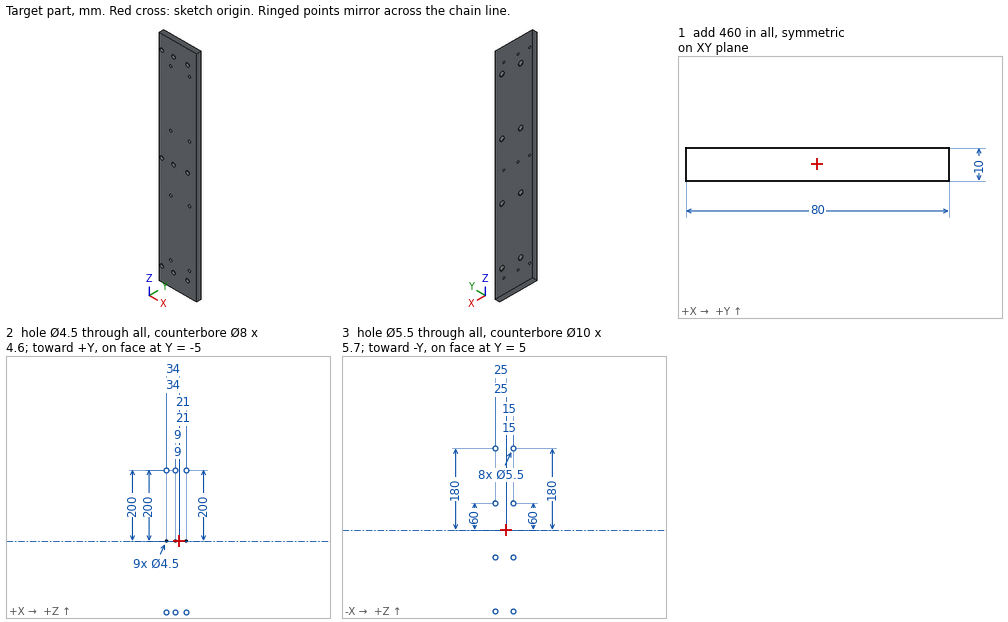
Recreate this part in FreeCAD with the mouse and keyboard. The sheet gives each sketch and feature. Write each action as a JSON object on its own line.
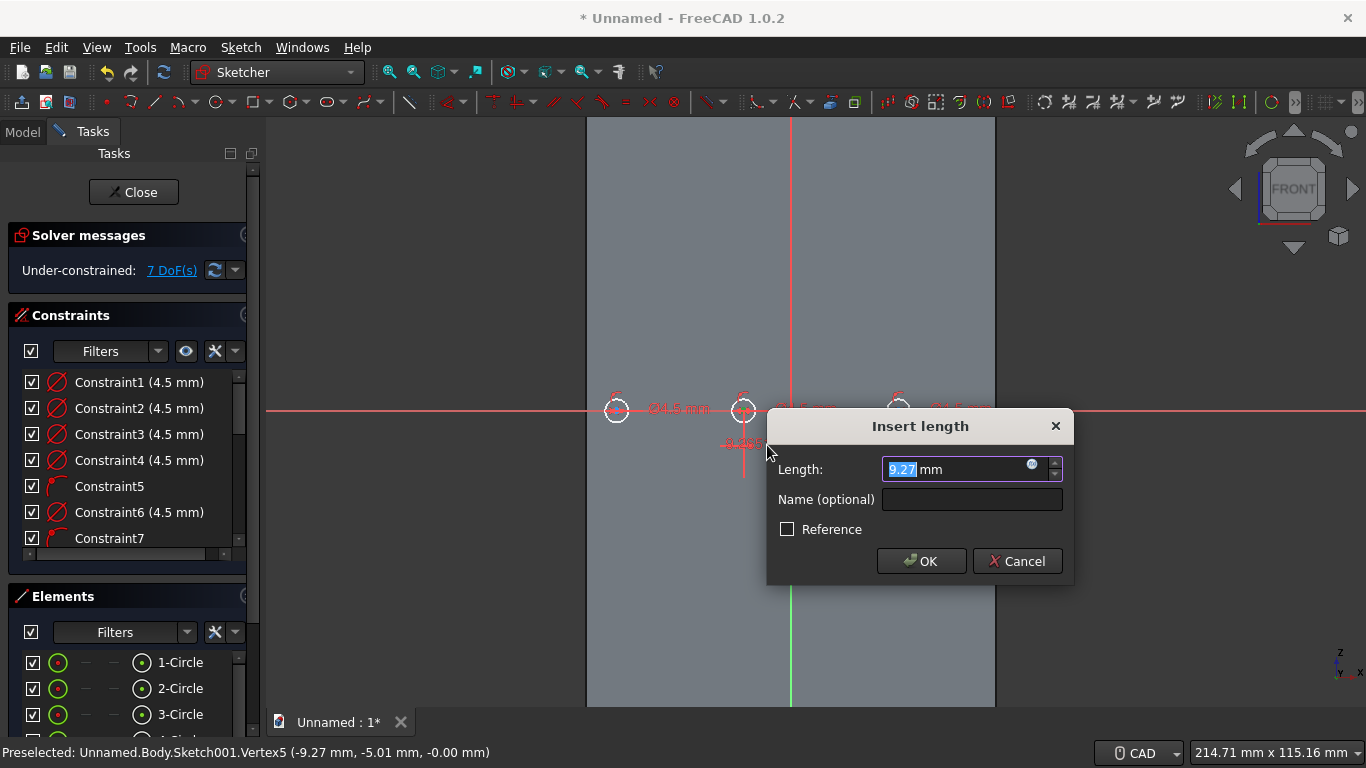
{"action": "type", "text": "9"}
{"action": "key", "text": "Return"}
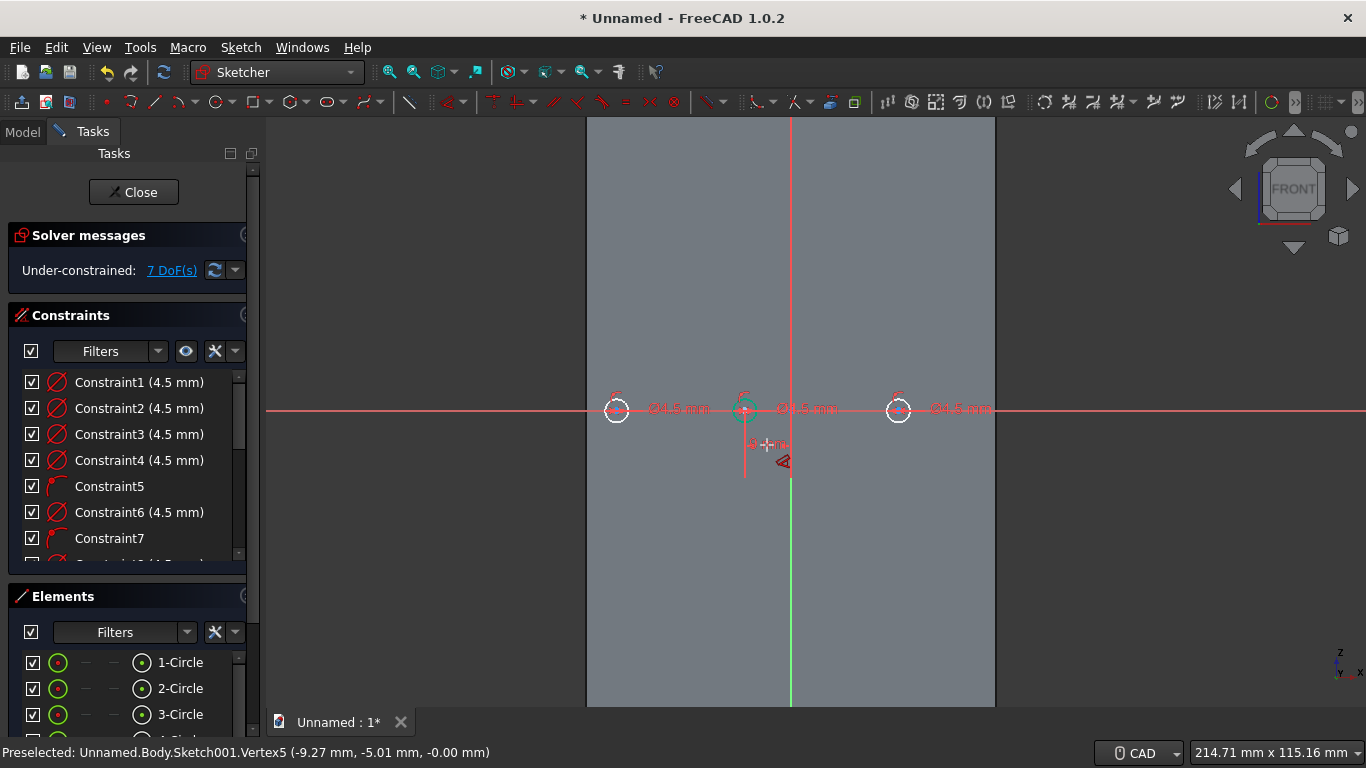
{"action": "scroll", "coordinate": [745, 412], "scroll_direction": "down", "scroll_amount": 9}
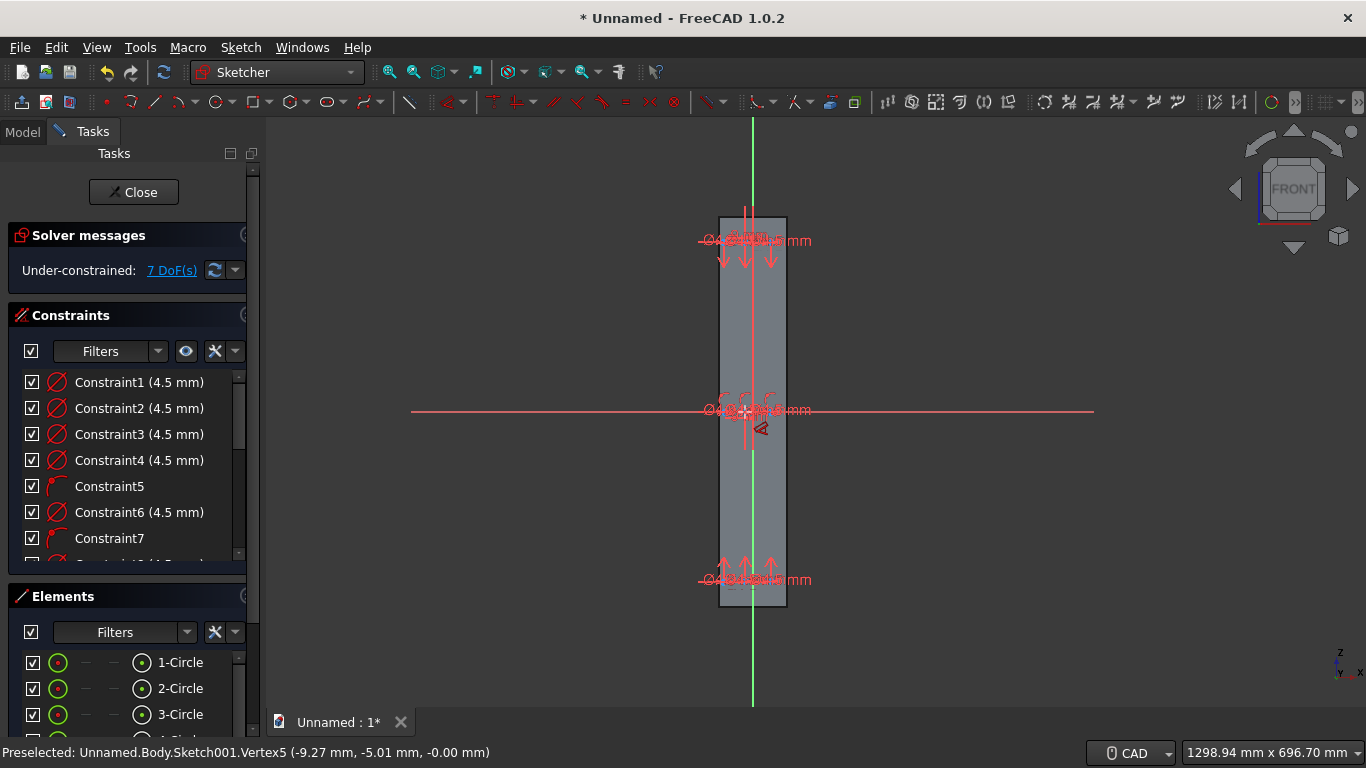
{"action": "scroll", "coordinate": [724, 242], "scroll_direction": "up", "scroll_amount": 2}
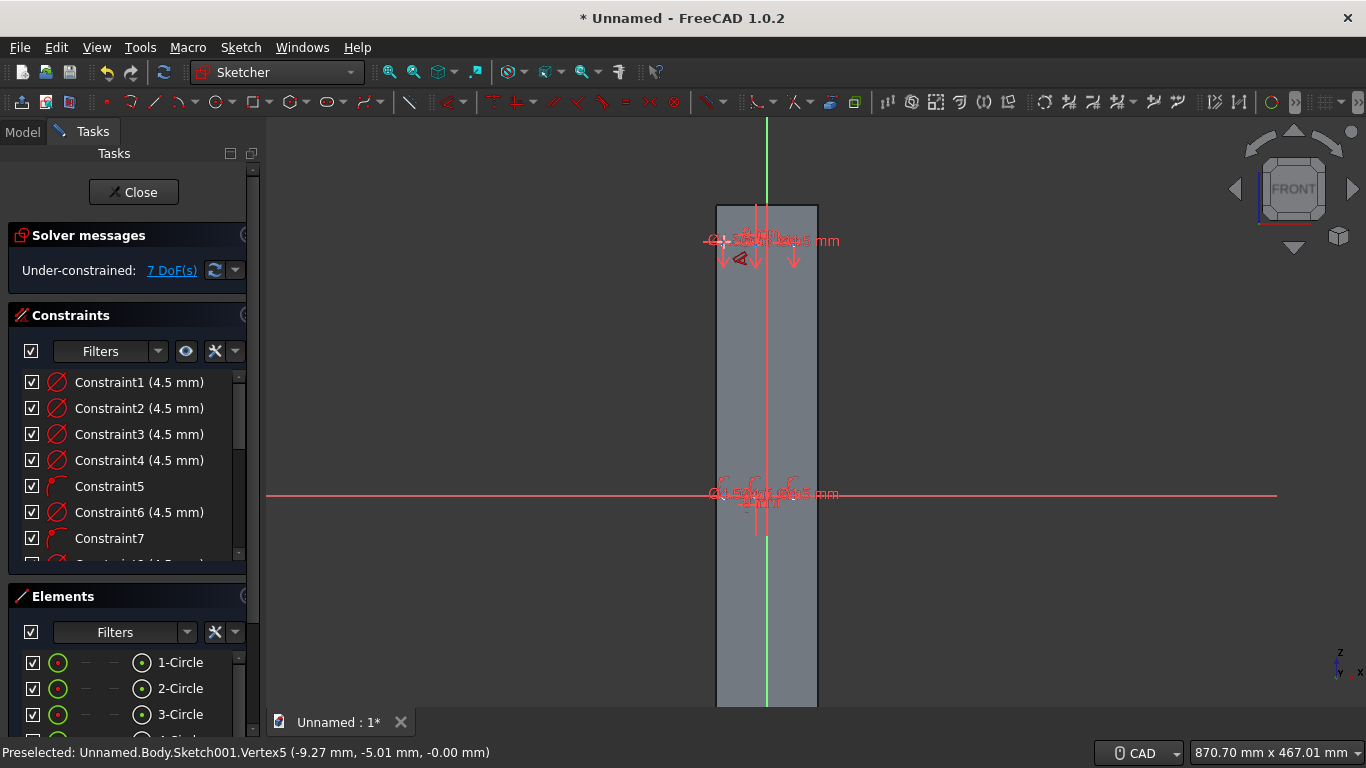
{"action": "left_click", "coordinate": [723, 242]}
{"action": "left_click", "coordinate": [745, 208]}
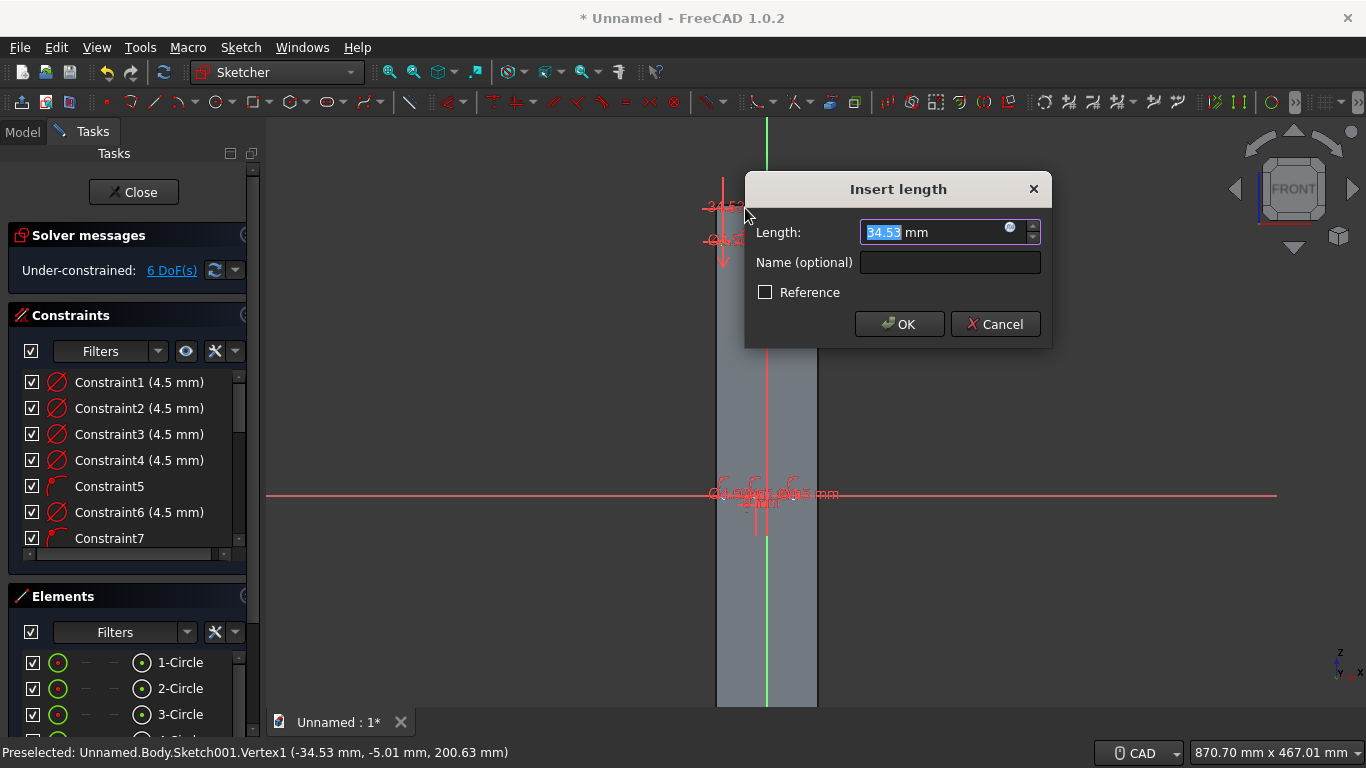
{"action": "type", "text": "34"}
{"action": "key", "text": "Return"}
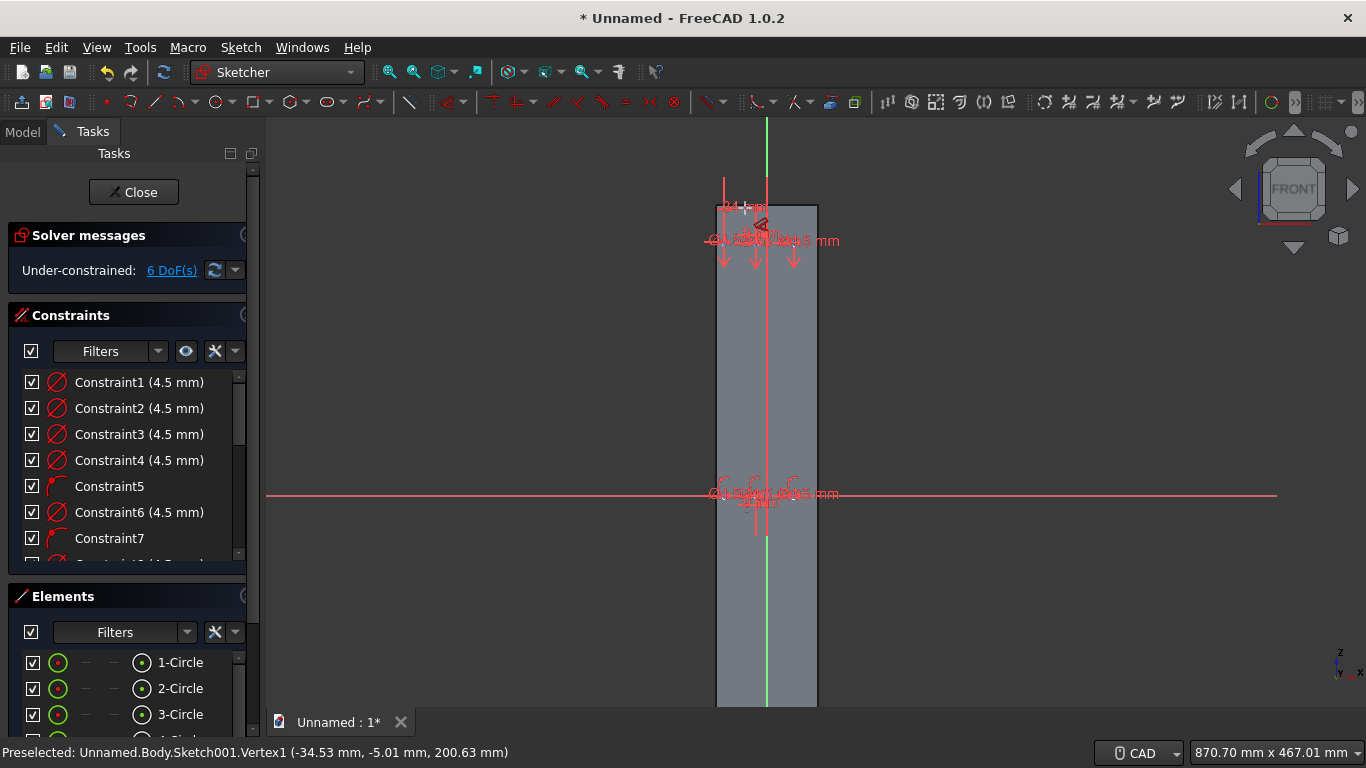
{"action": "scroll", "coordinate": [794, 243], "scroll_direction": "up", "scroll_amount": 3}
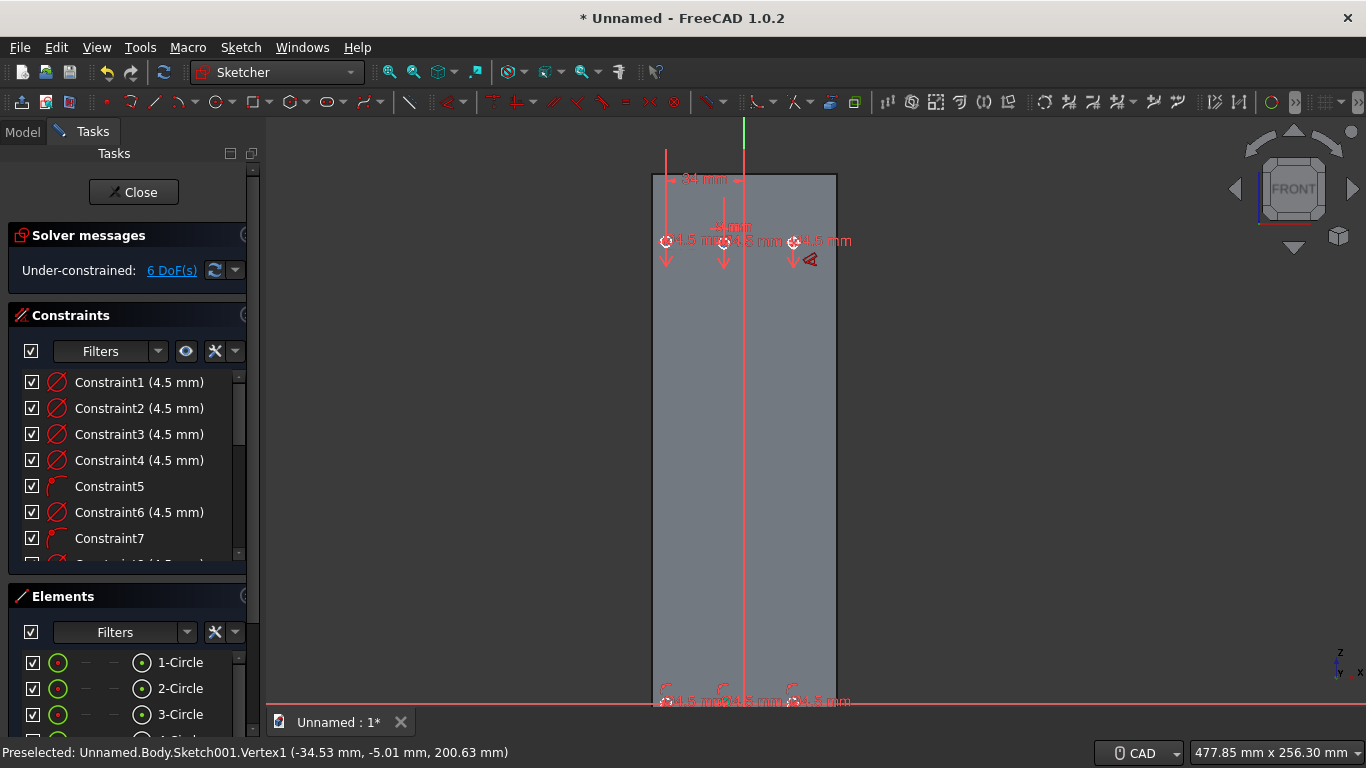
{"action": "left_click", "coordinate": [793, 243]}
{"action": "left_click", "coordinate": [780, 185]}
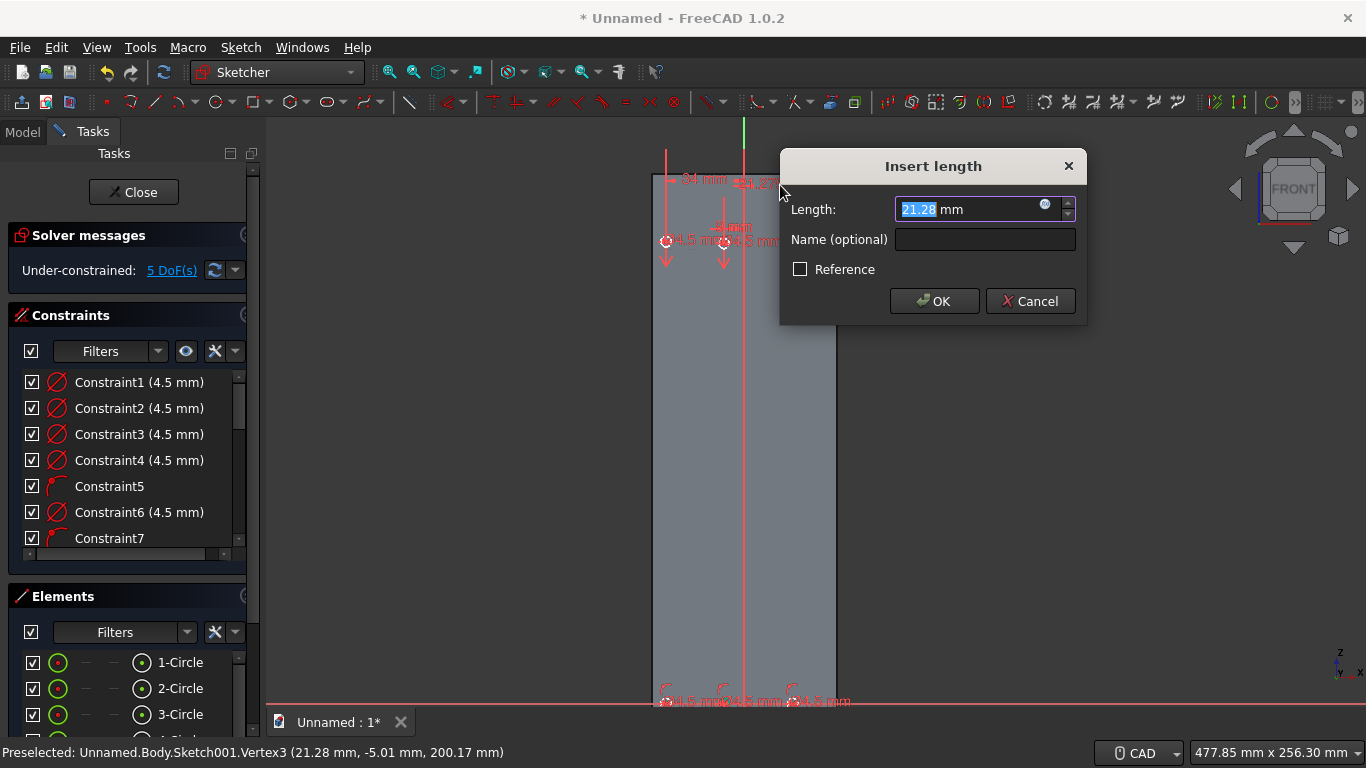
{"action": "type", "text": "21"}
{"action": "key", "text": "Return"}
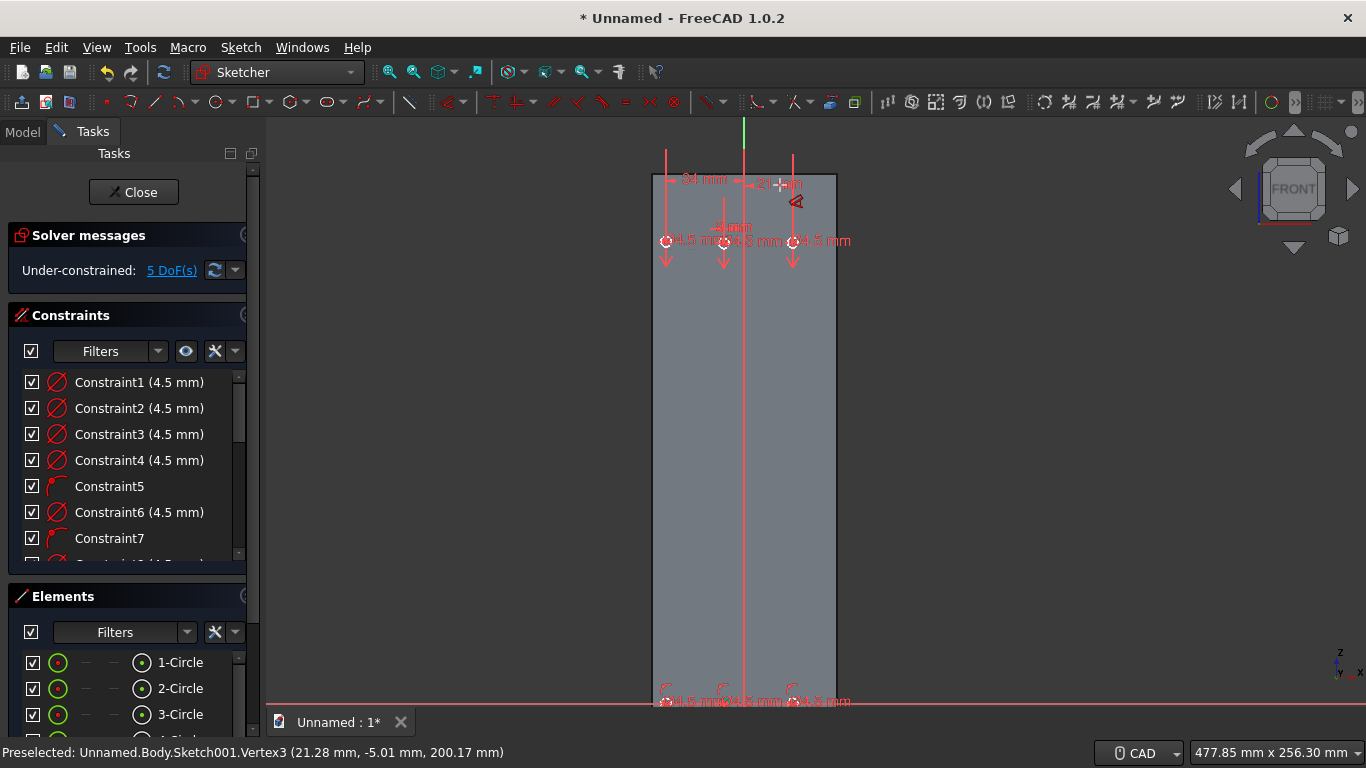
{"action": "scroll", "coordinate": [758, 242], "scroll_direction": "down", "scroll_amount": 5}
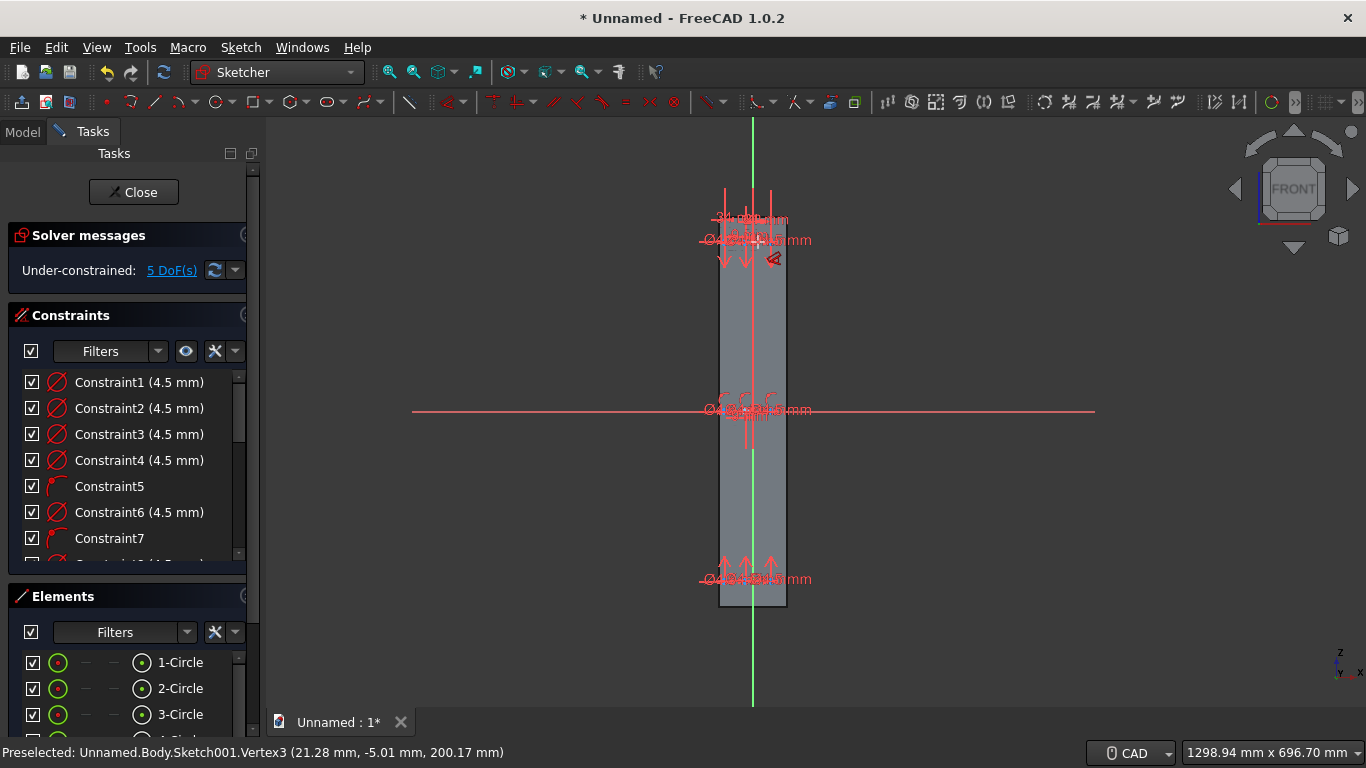
{"action": "scroll", "coordinate": [725, 412], "scroll_direction": "up", "scroll_amount": 2}